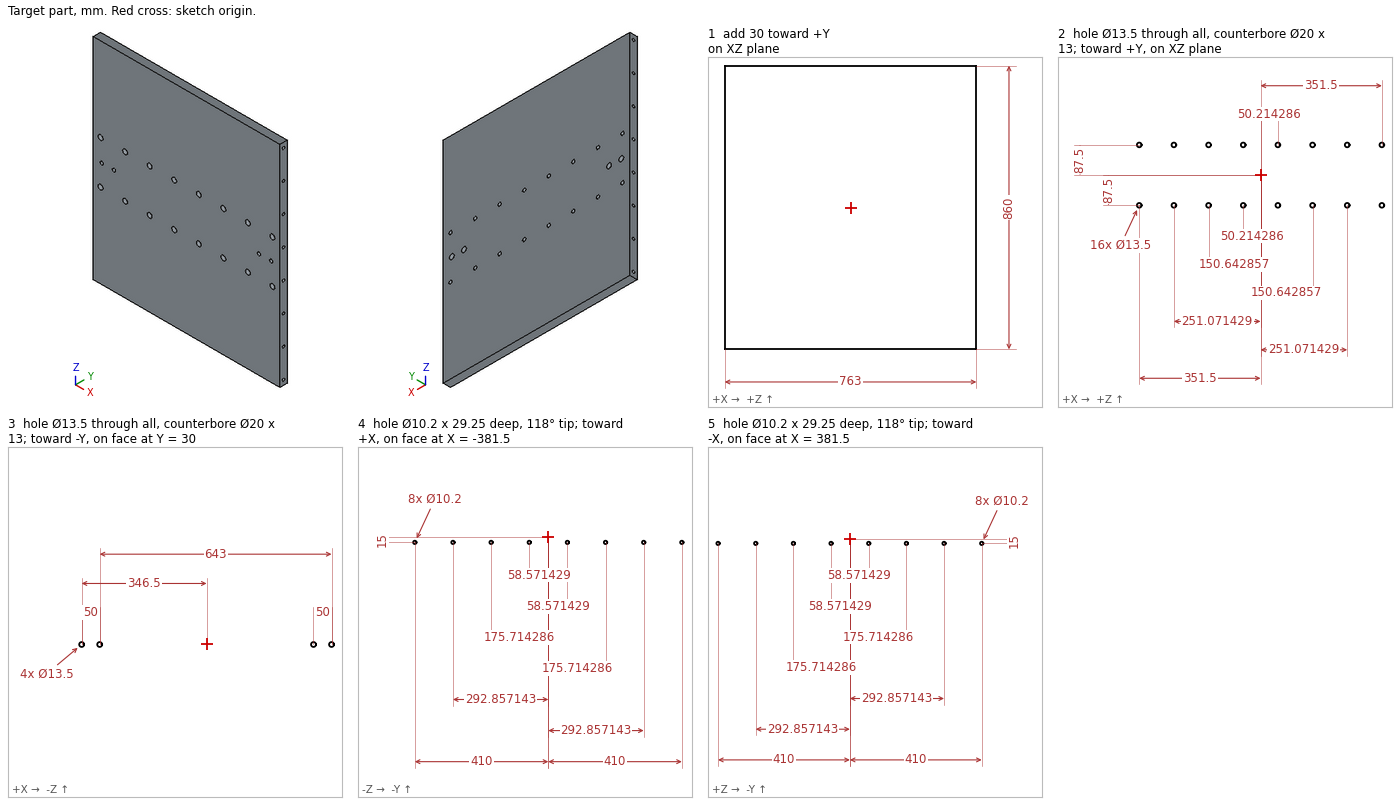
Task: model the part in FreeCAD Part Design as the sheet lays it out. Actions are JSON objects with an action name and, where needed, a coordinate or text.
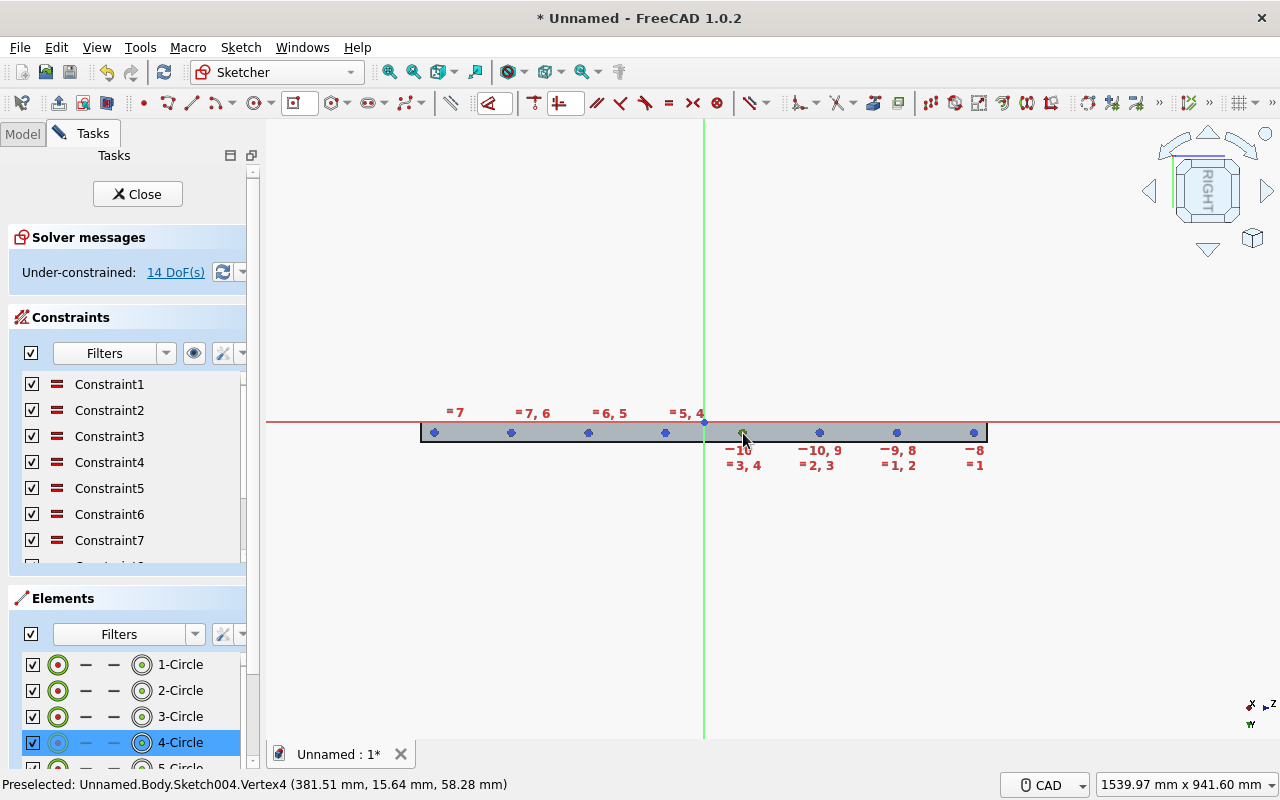
{"action": "left_click", "coordinate": [666, 433]}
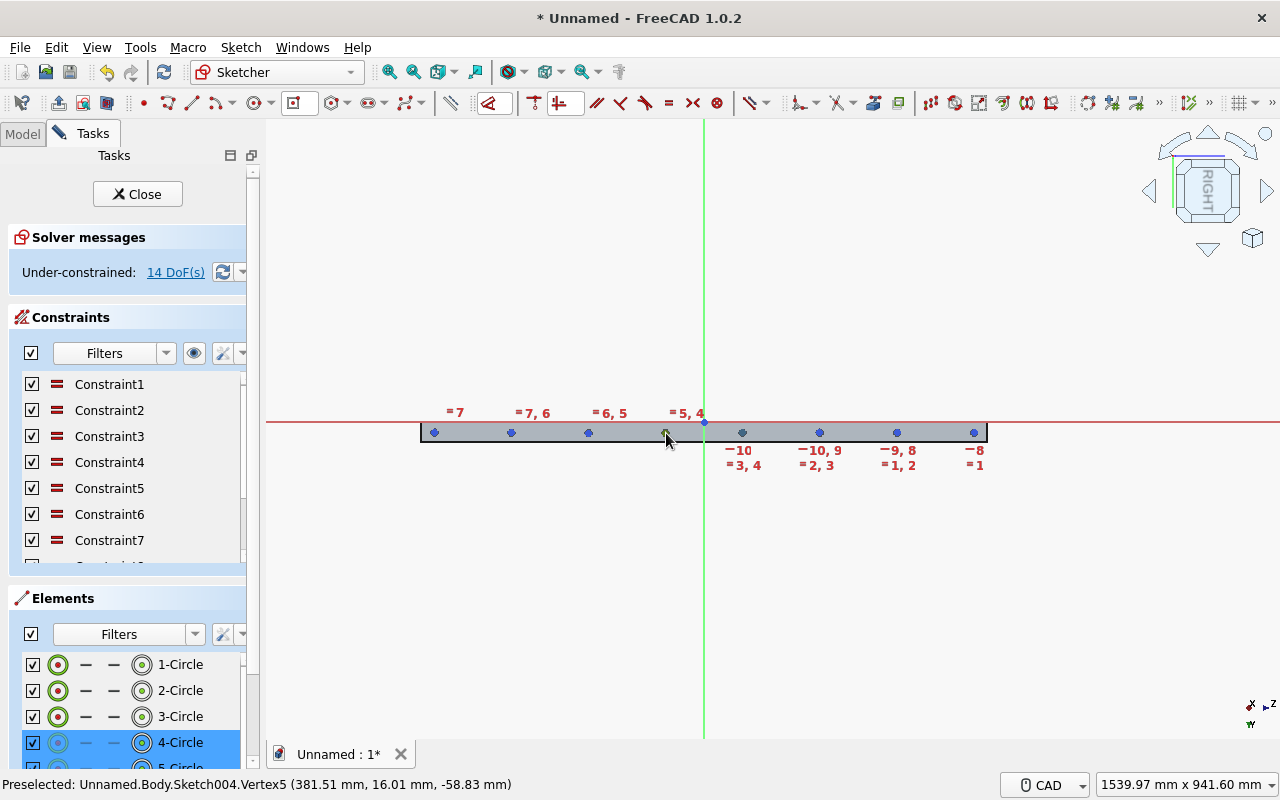
{"action": "key", "text": "h"}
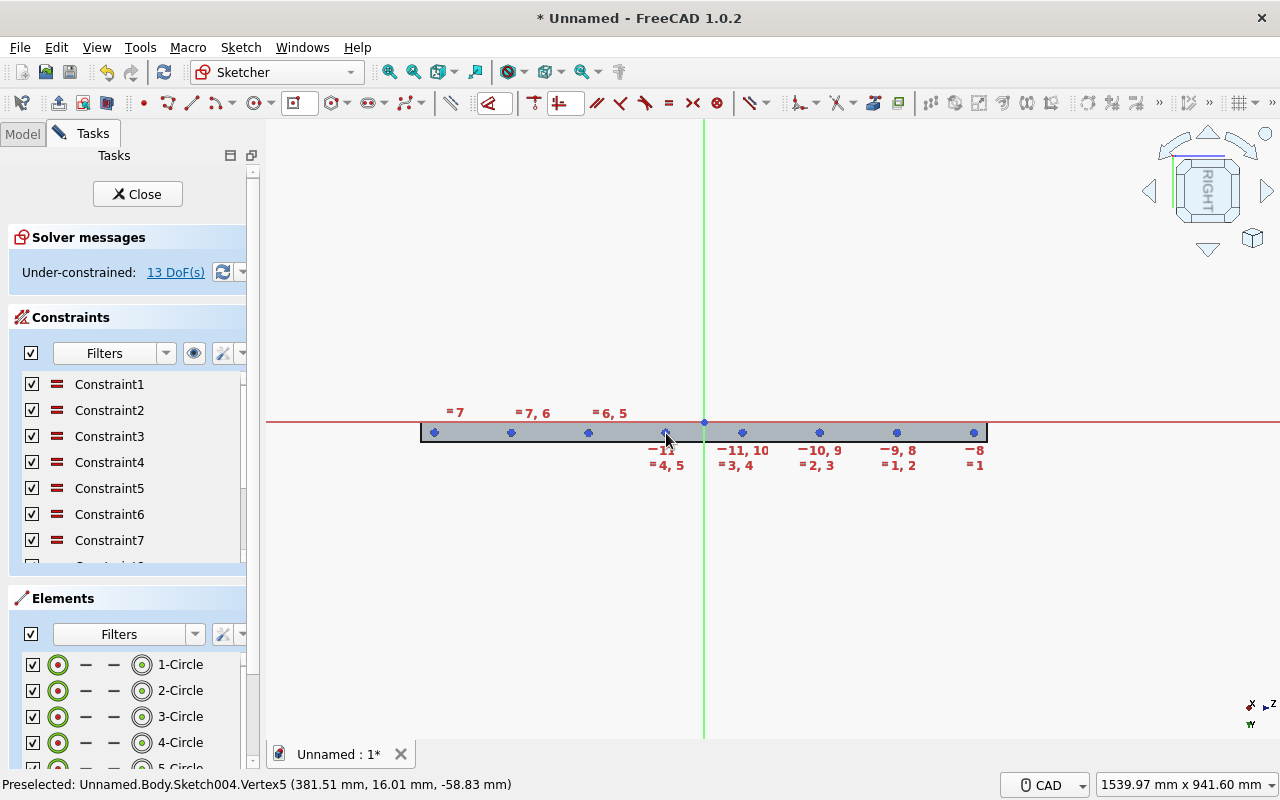
{"action": "left_click", "coordinate": [666, 433]}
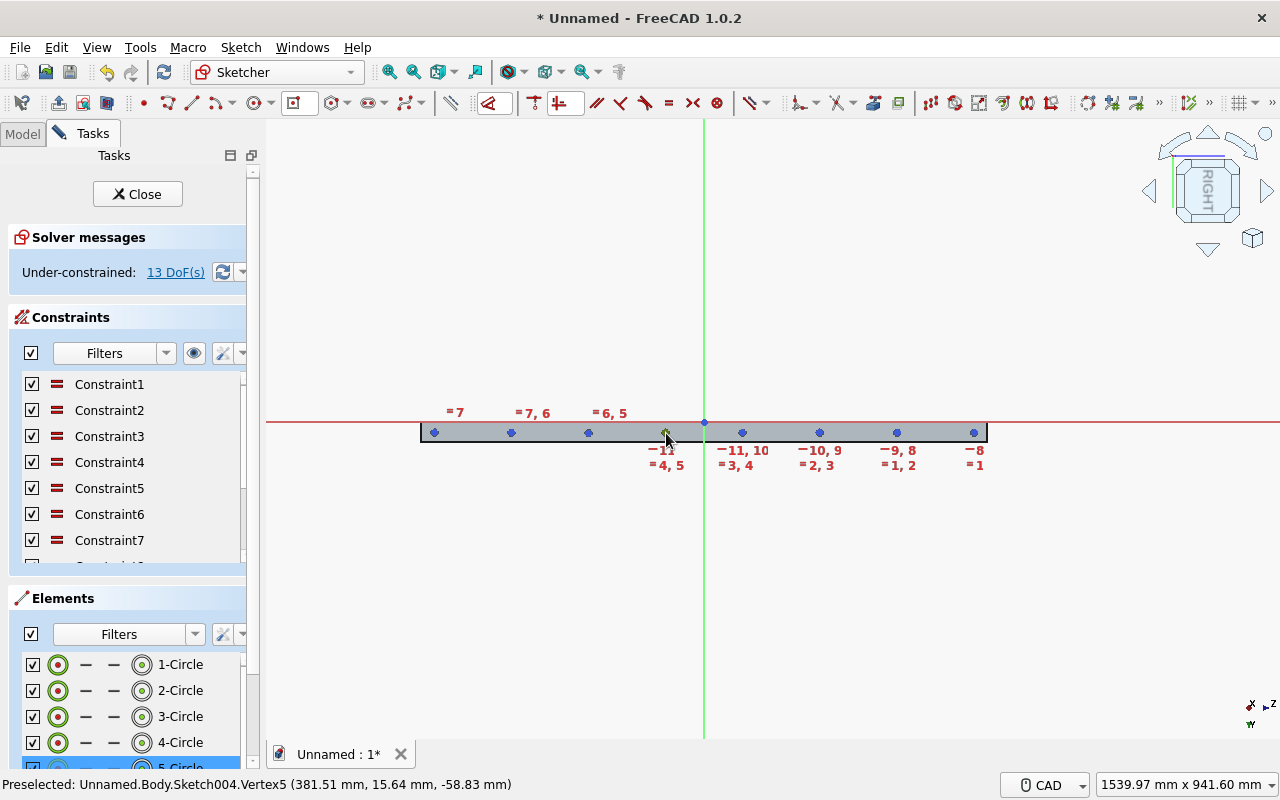
{"action": "left_click", "coordinate": [589, 433]}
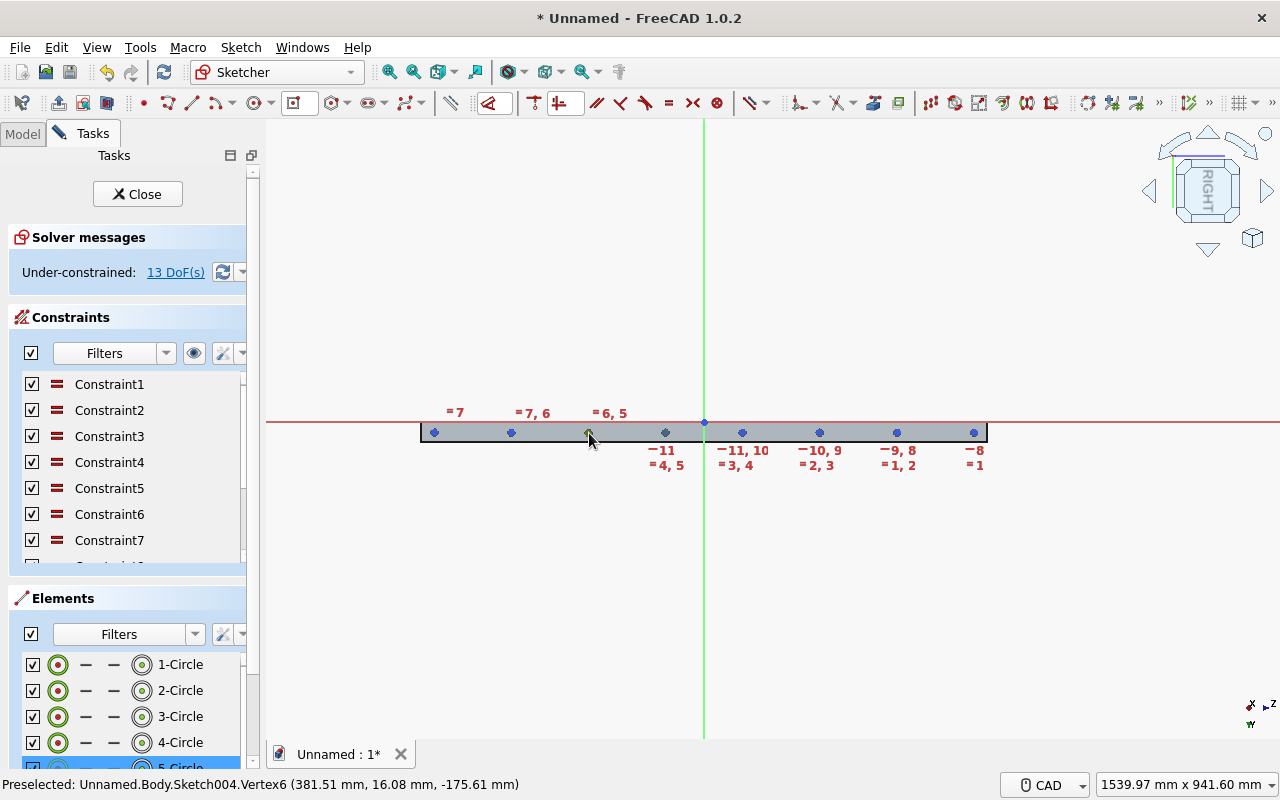
{"action": "left_click", "coordinate": [578, 104]}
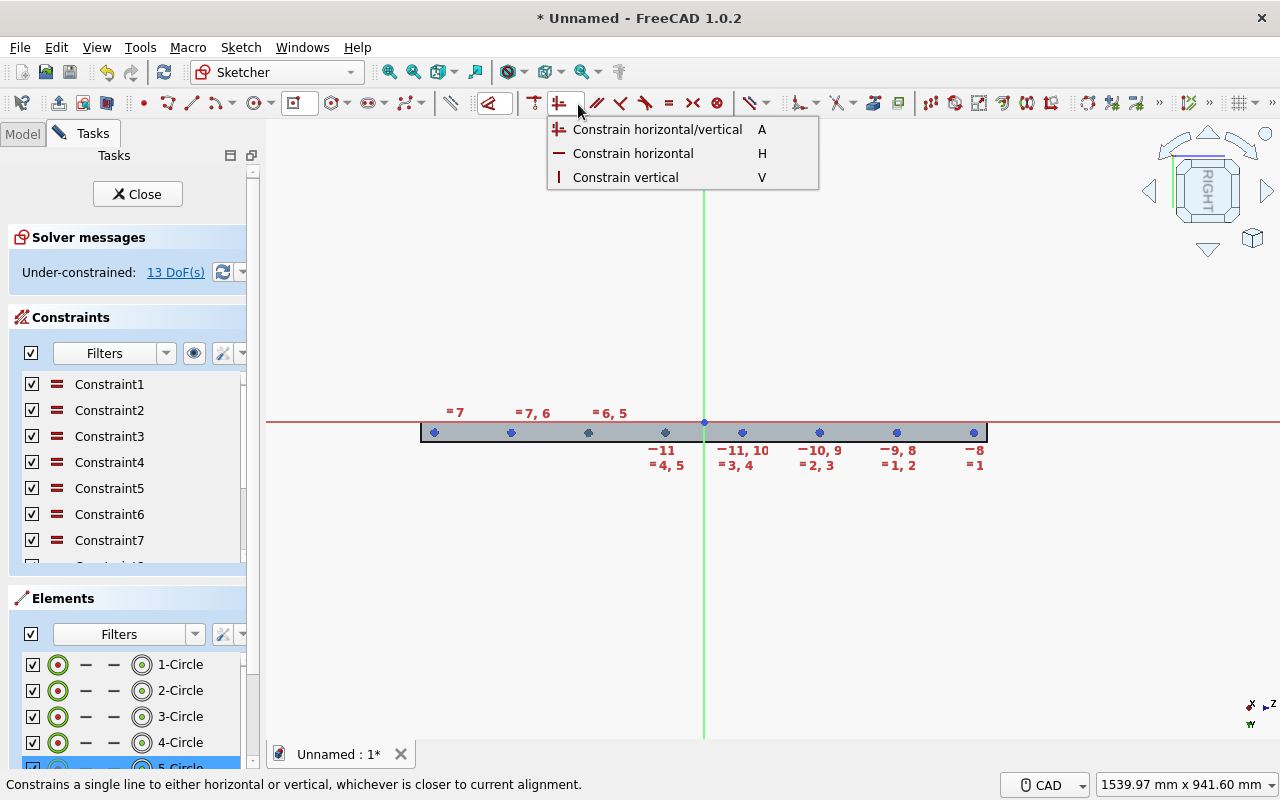
{"action": "left_click", "coordinate": [683, 153]}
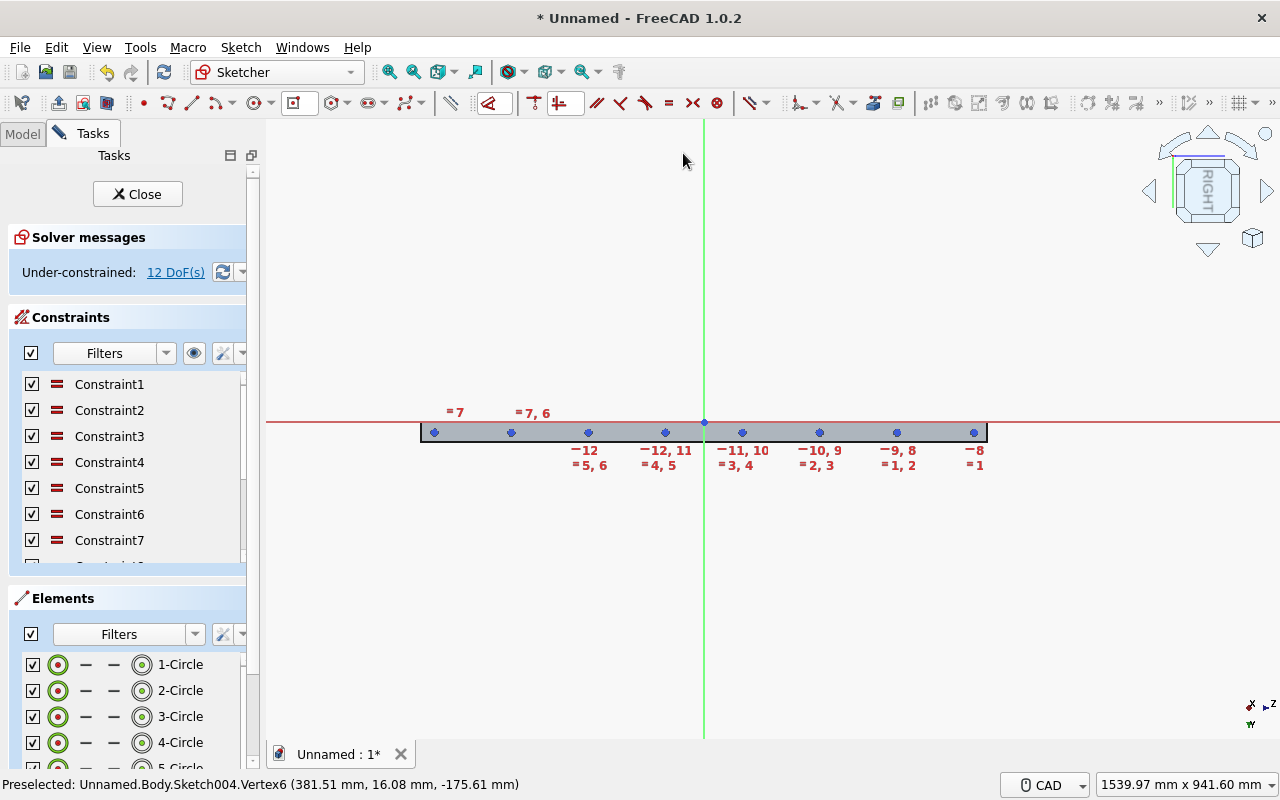
{"action": "left_click", "coordinate": [589, 433]}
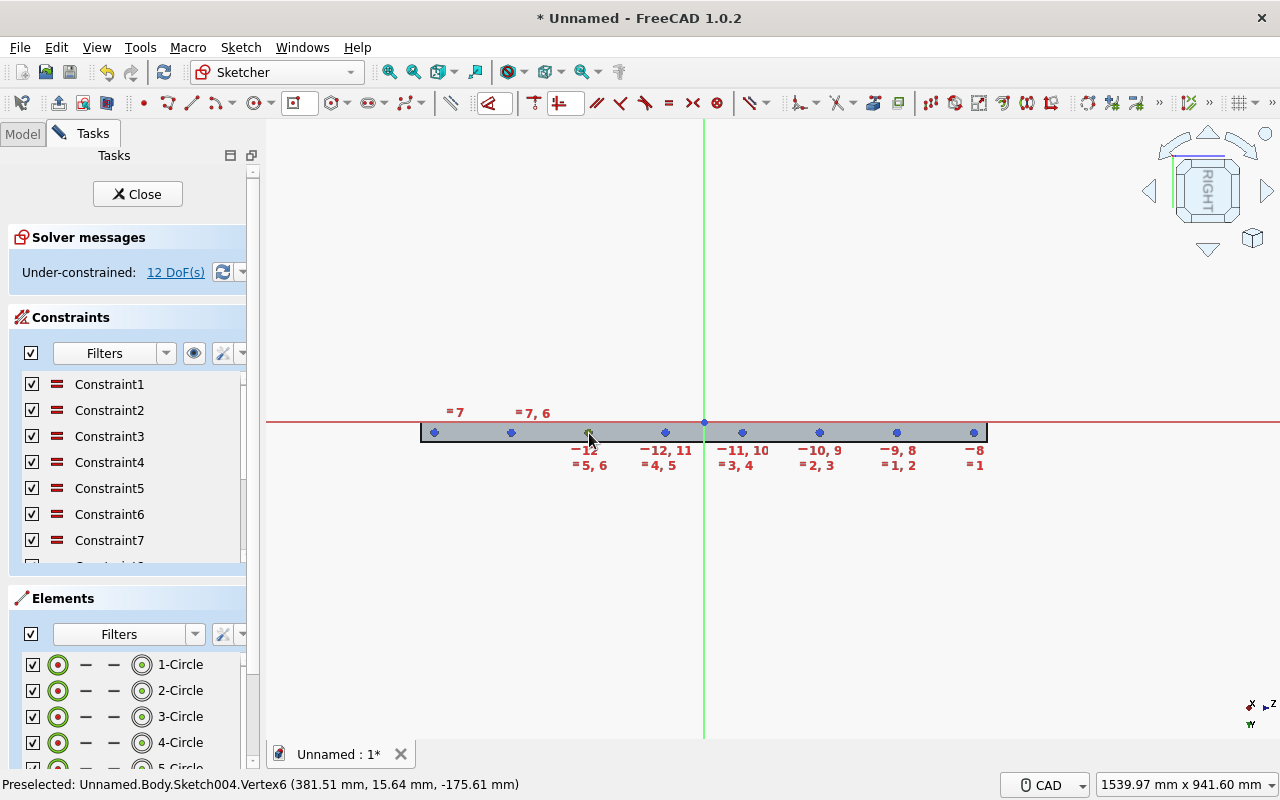
{"action": "left_click", "coordinate": [511, 433]}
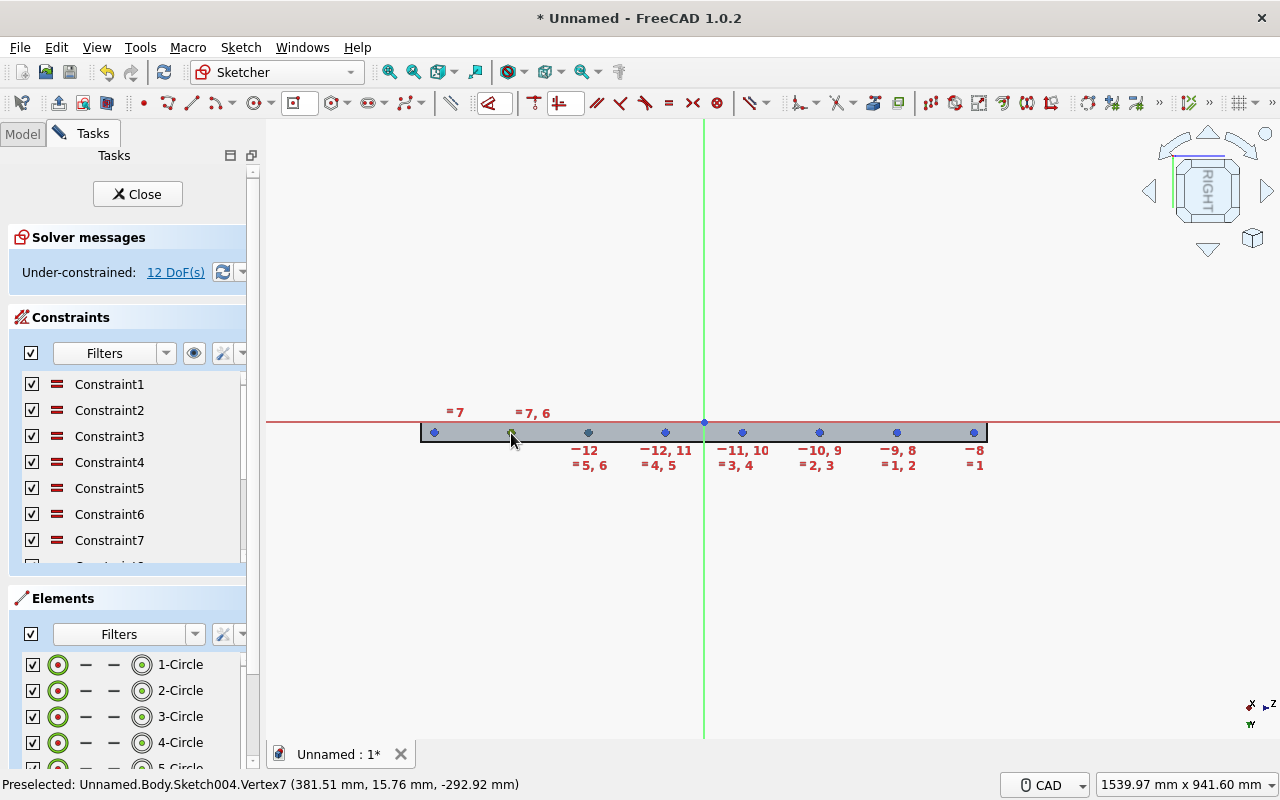
{"action": "key", "text": "h"}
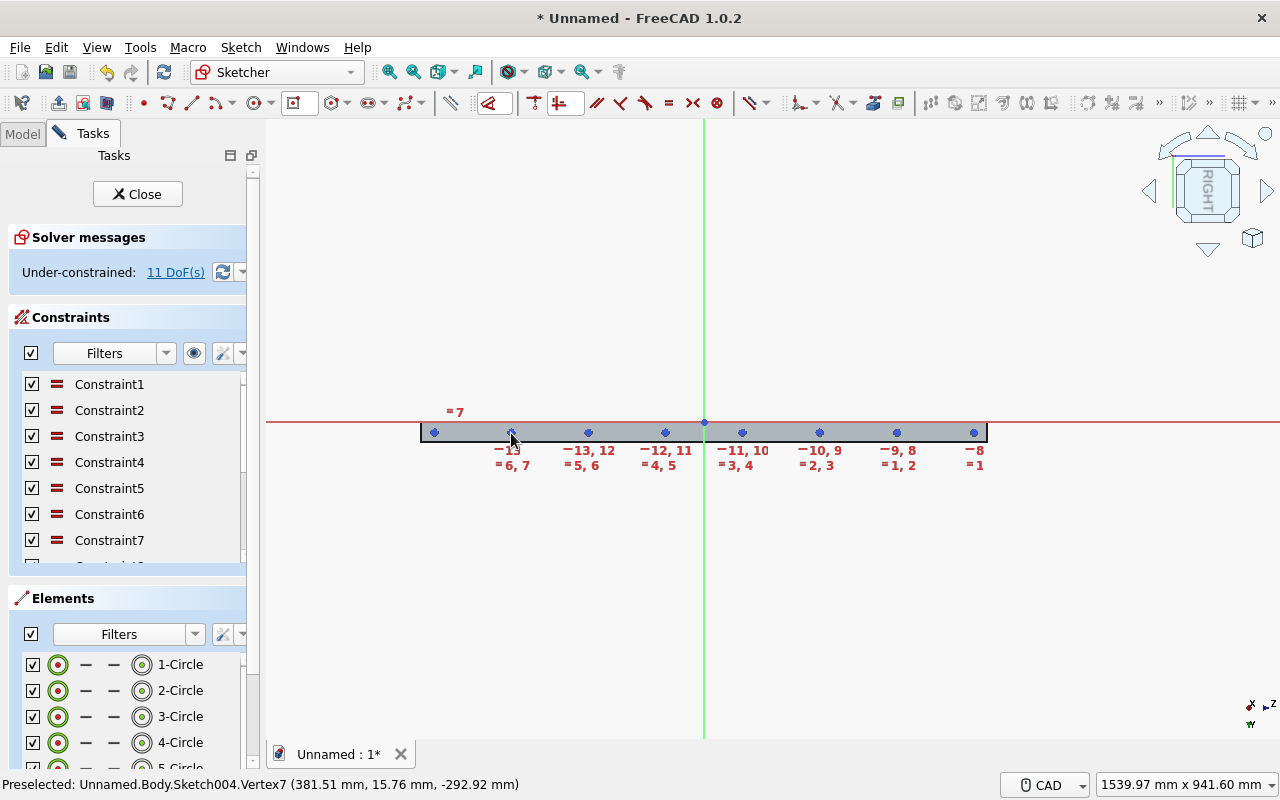
{"action": "left_click", "coordinate": [511, 433]}